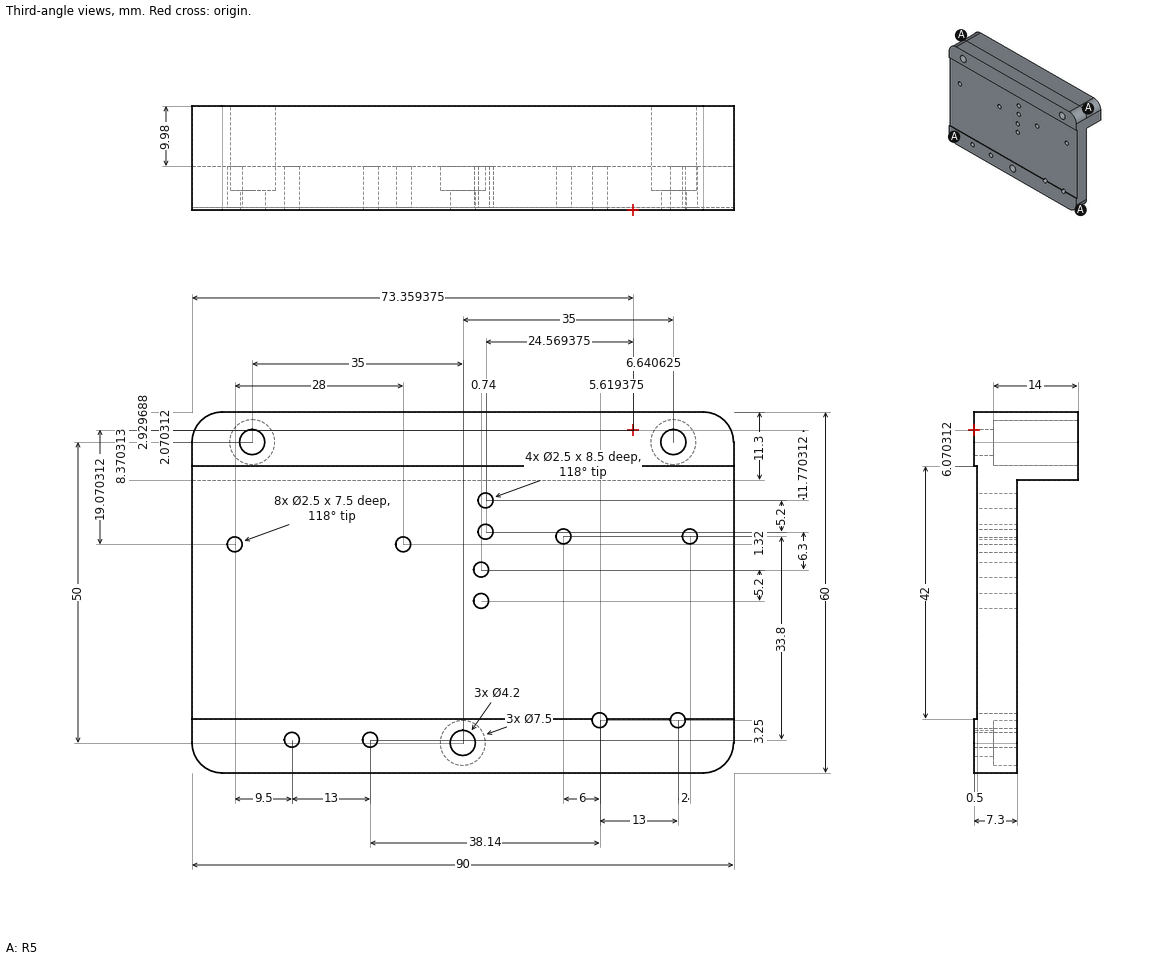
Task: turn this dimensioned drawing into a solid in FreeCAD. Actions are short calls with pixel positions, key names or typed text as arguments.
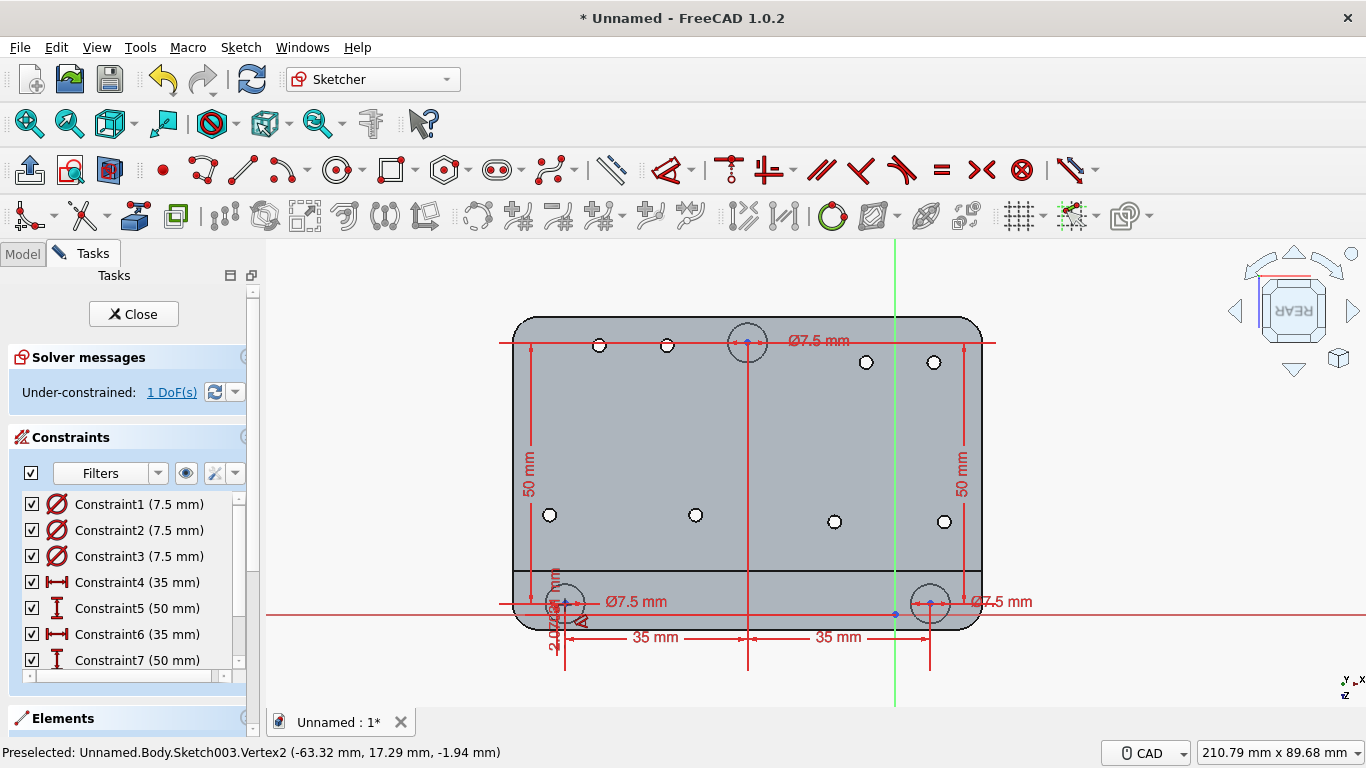
click(930, 604)
click(913, 649)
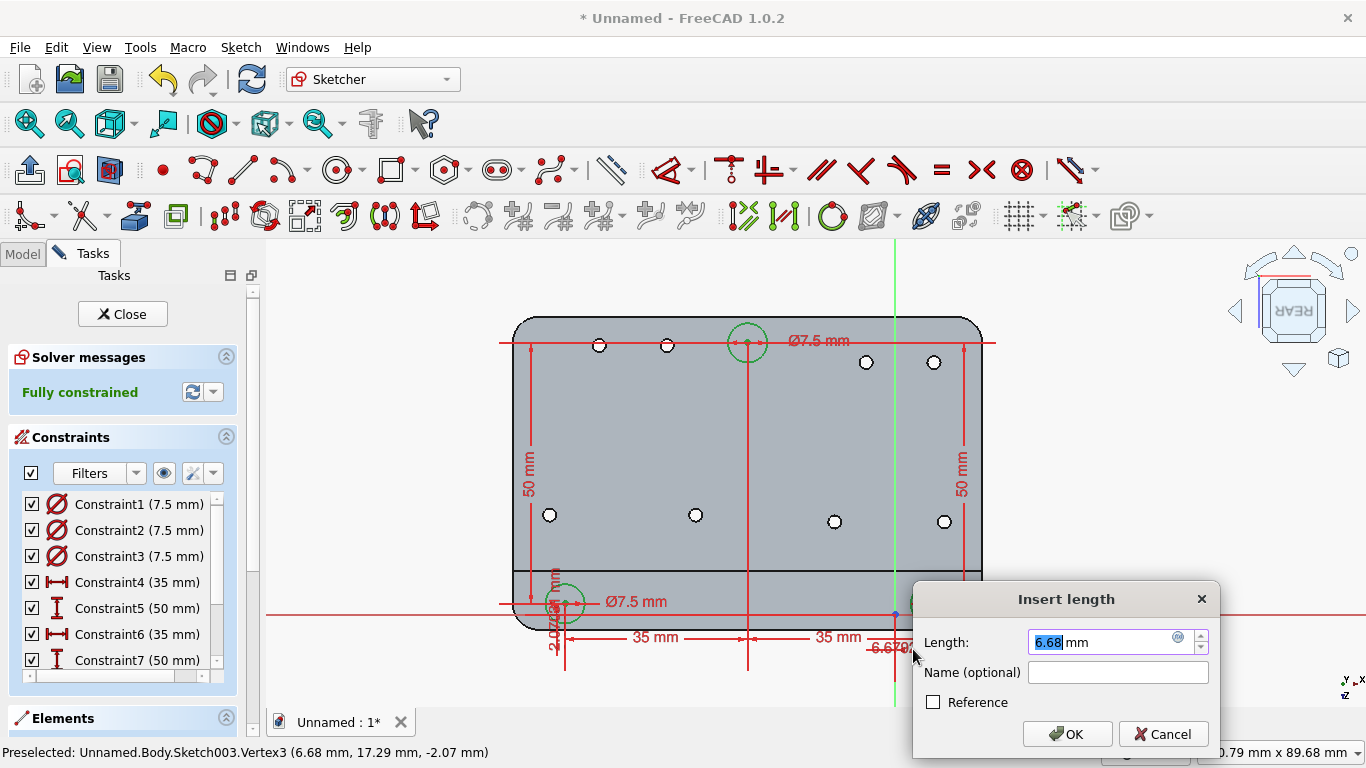
text(6.640625)
key(Return)
key(Escape)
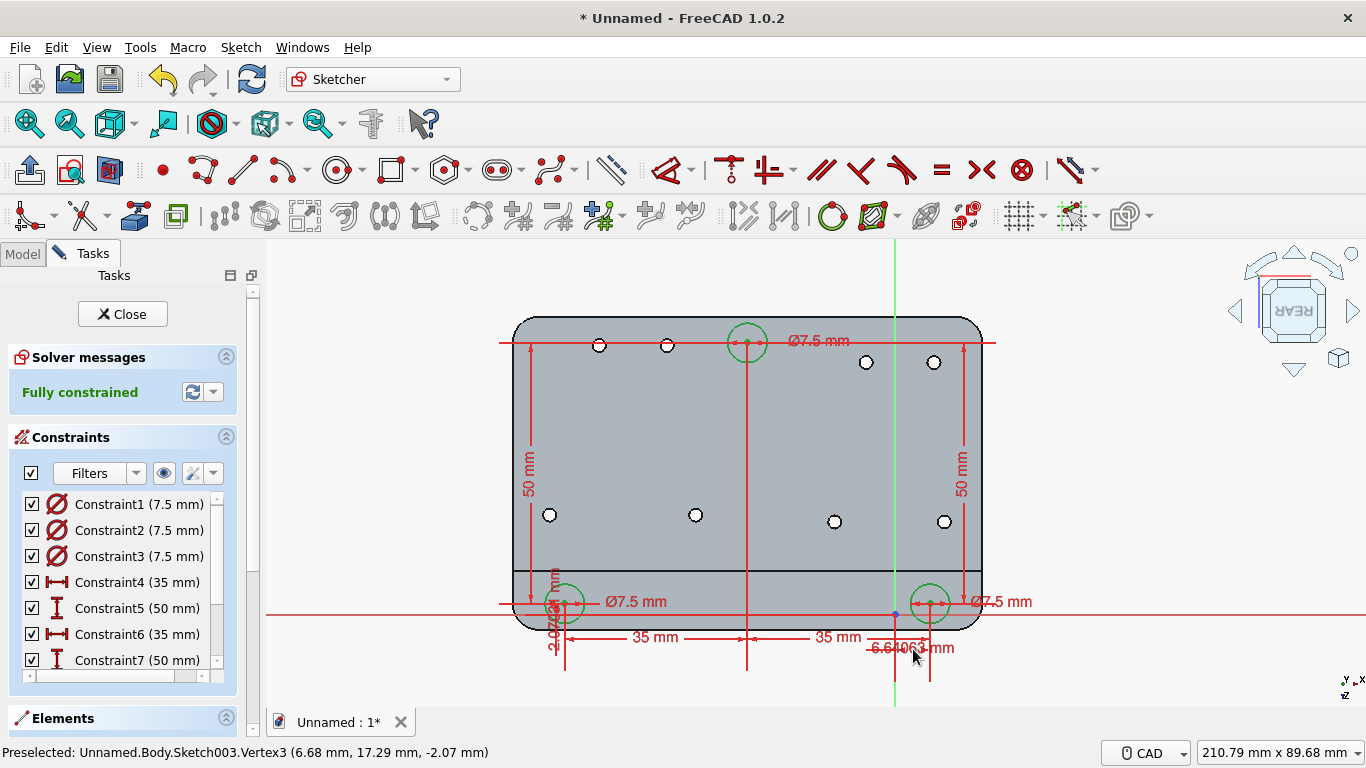
click(123, 314)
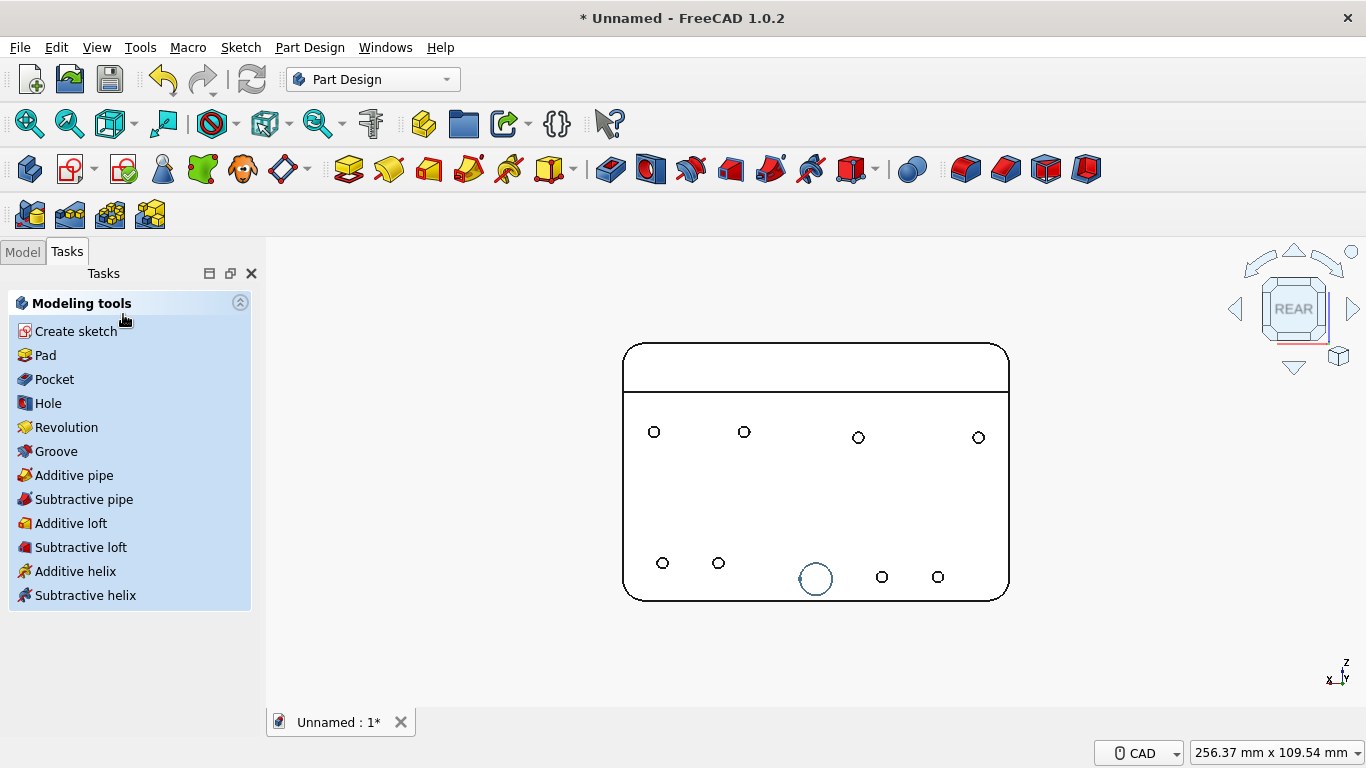
click(612, 170)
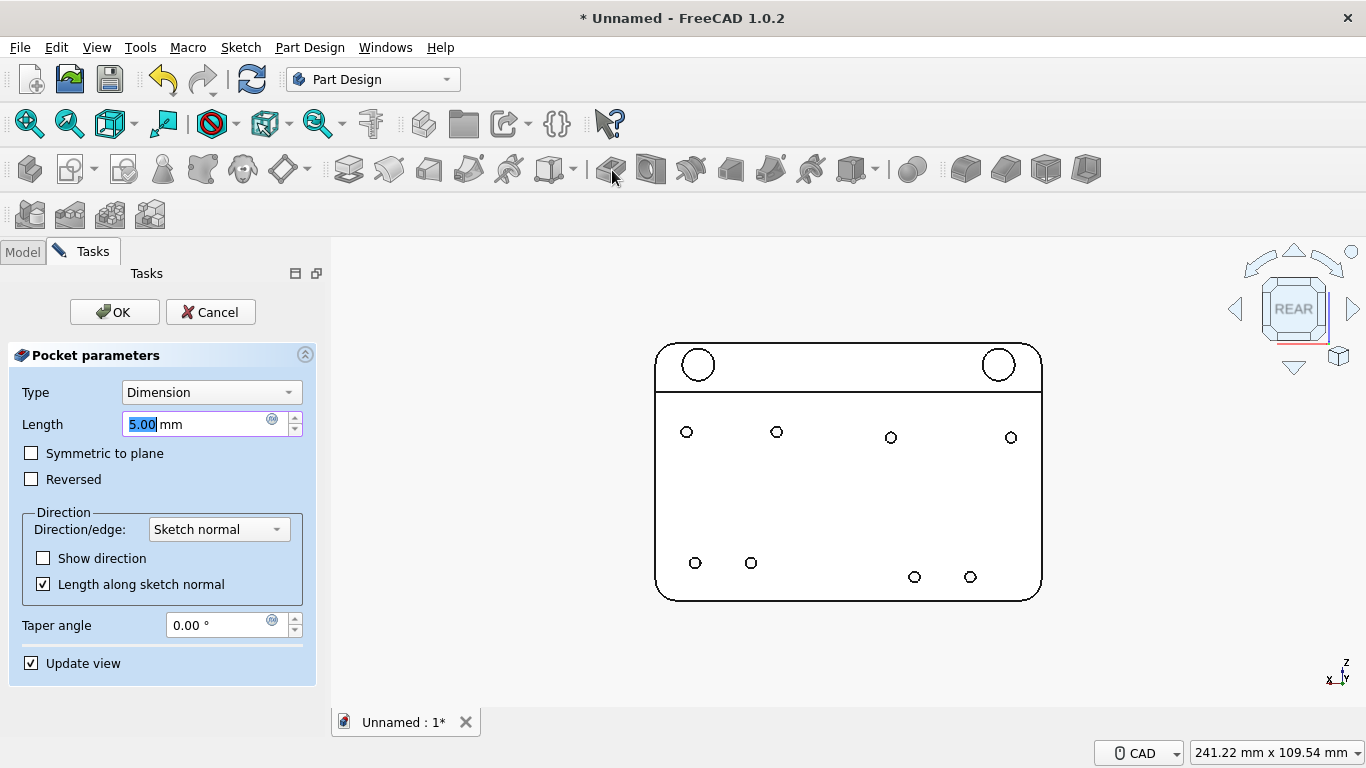
text(14)
key(Tab)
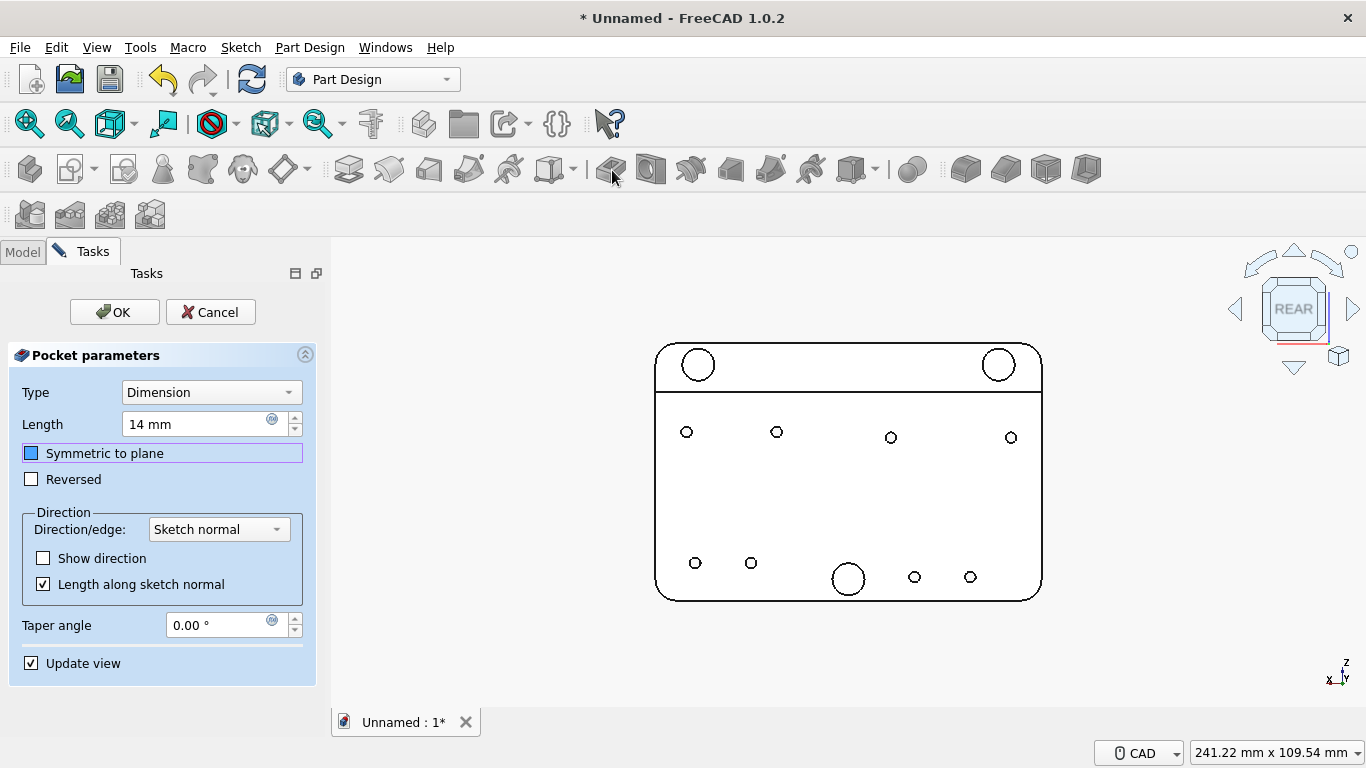
click(115, 312)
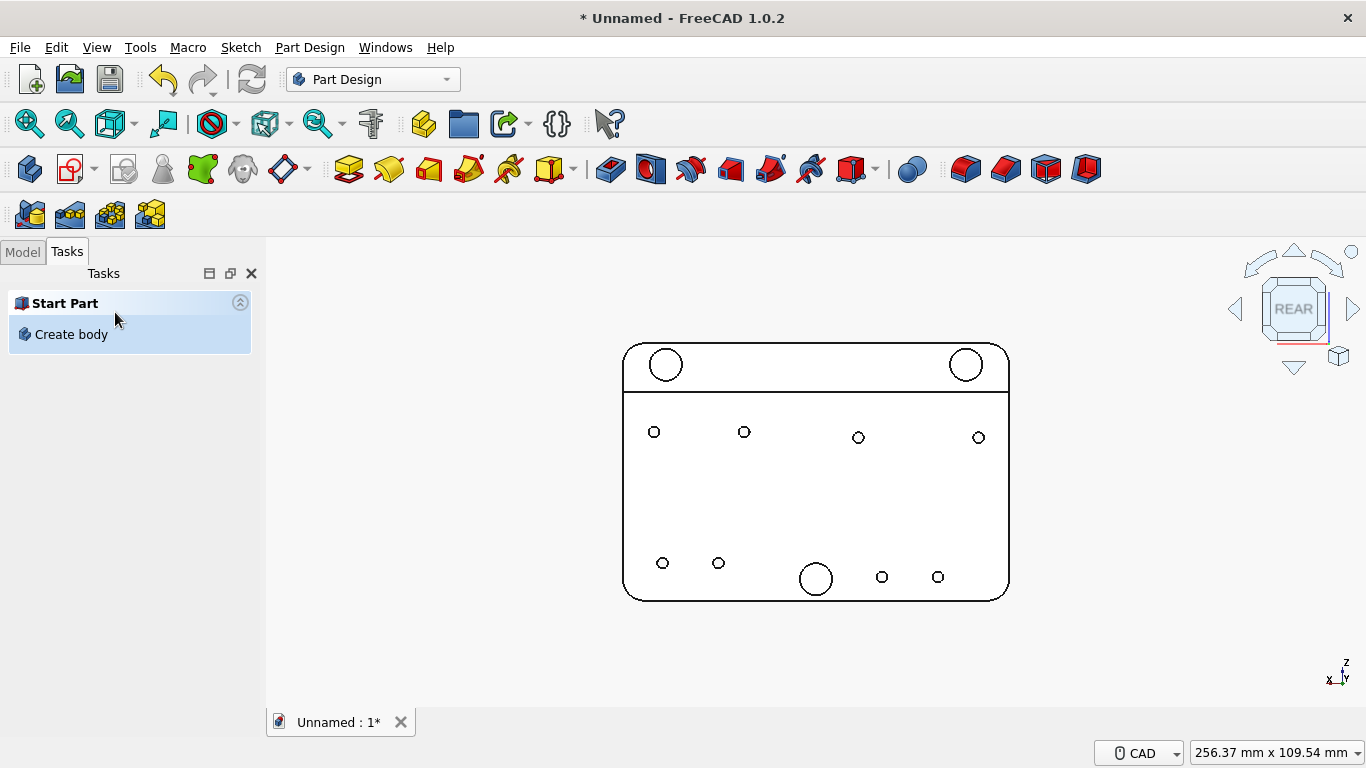
click(666, 364)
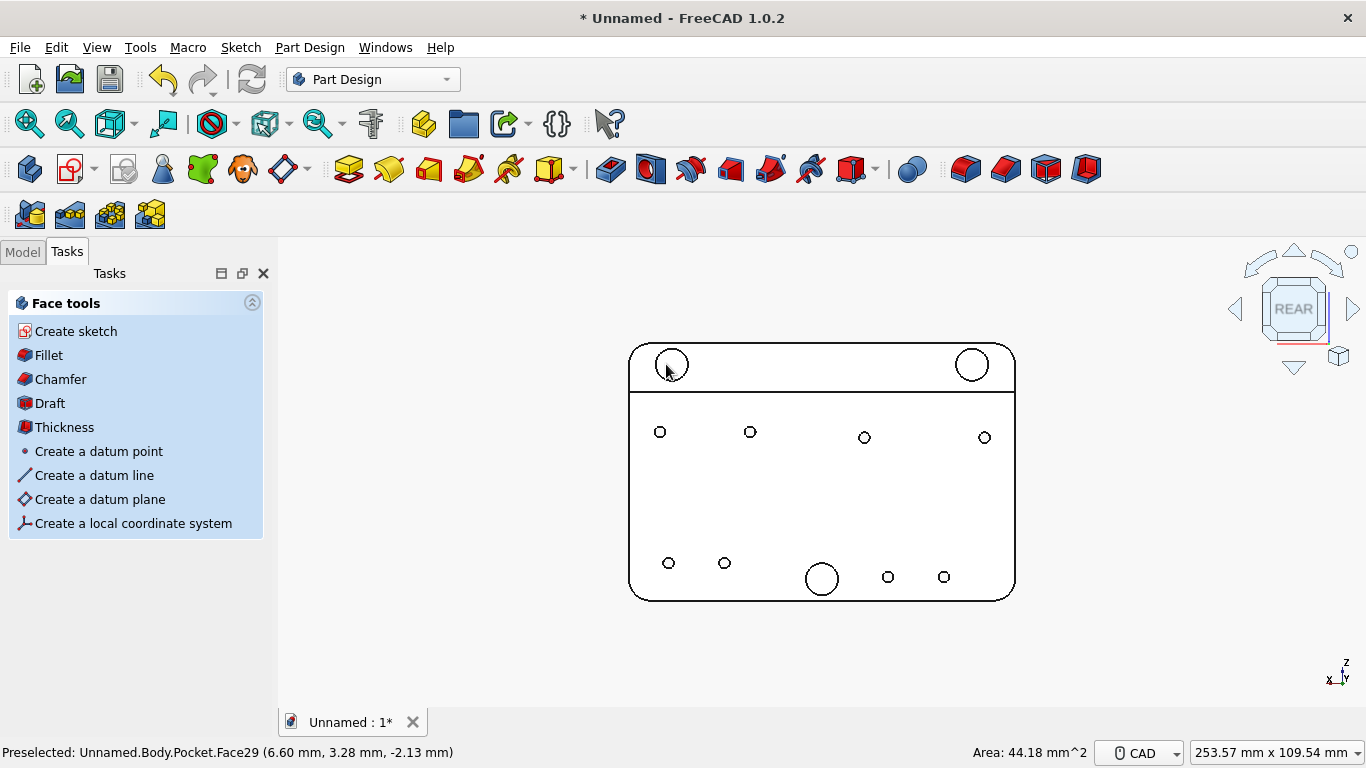
click(70, 170)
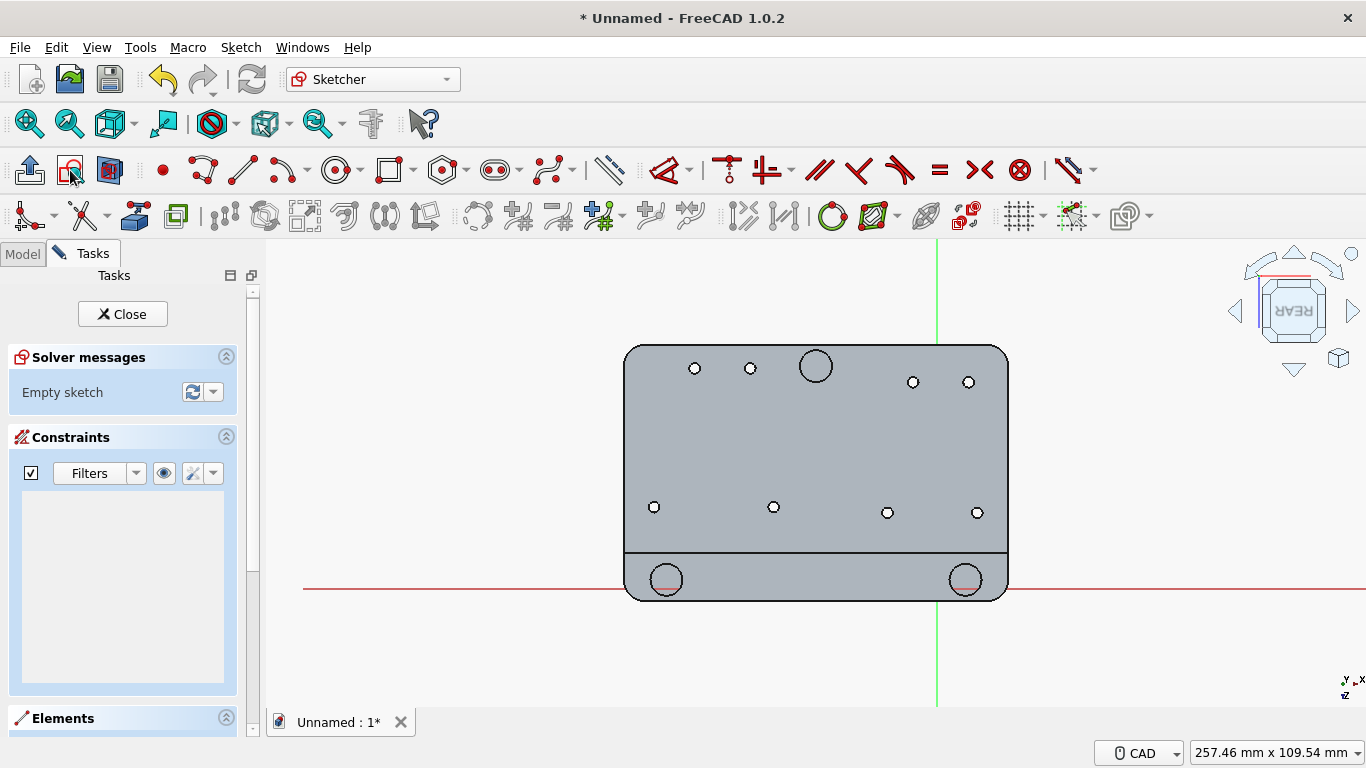
click(336, 170)